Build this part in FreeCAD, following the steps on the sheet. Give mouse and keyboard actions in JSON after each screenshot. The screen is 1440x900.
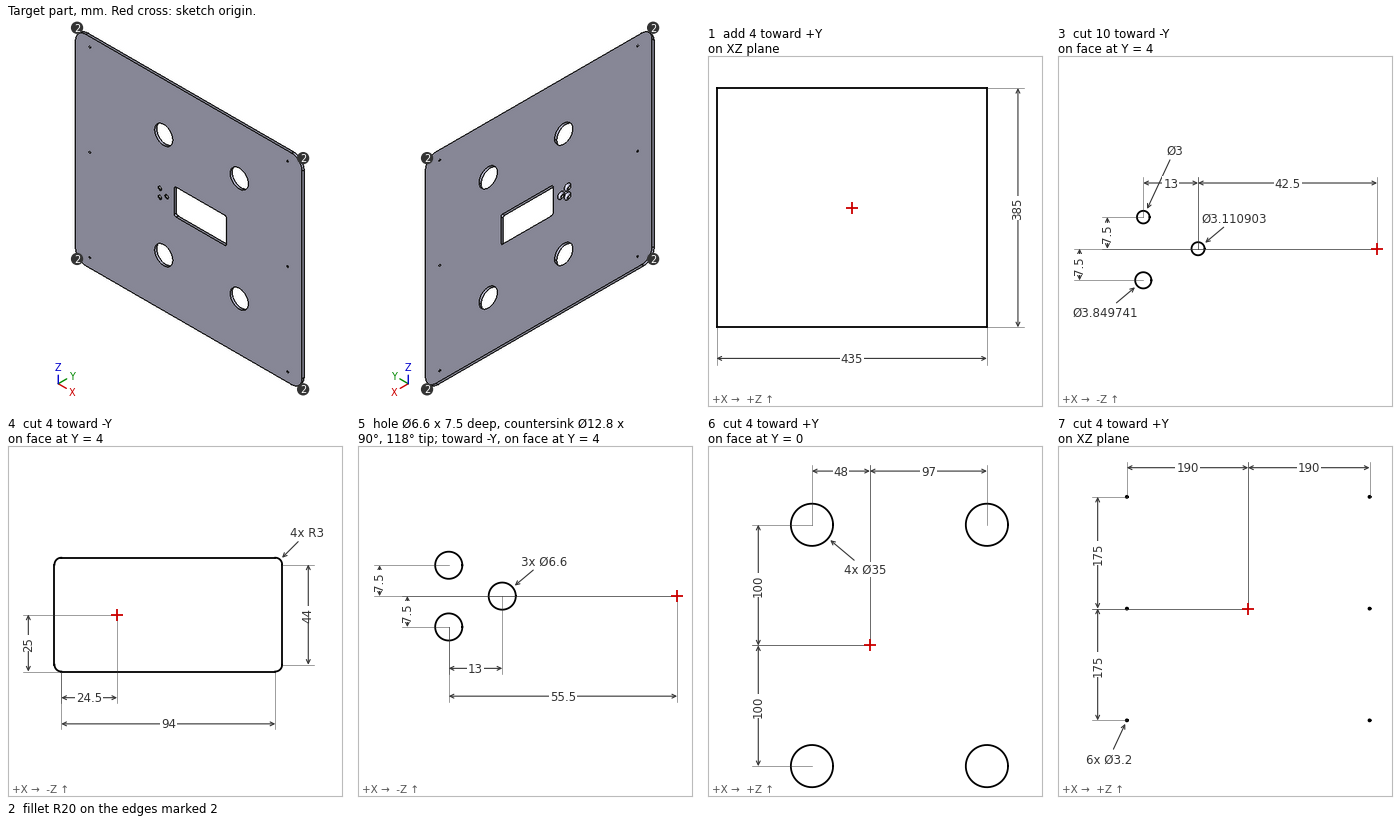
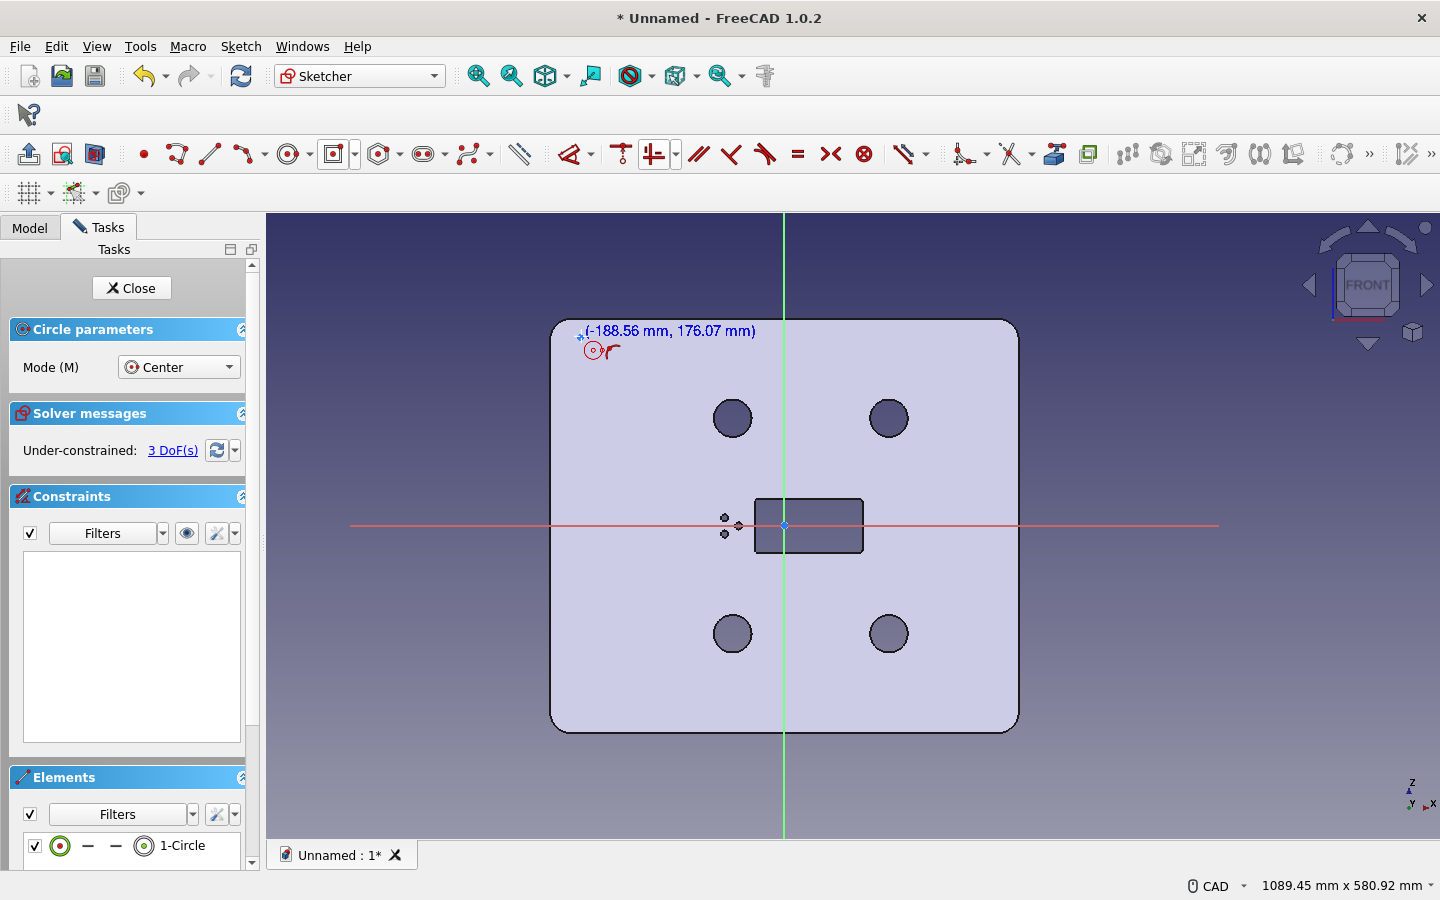
{"action": "scroll", "coordinate": [580, 526], "scroll_direction": "up", "scroll_amount": 13}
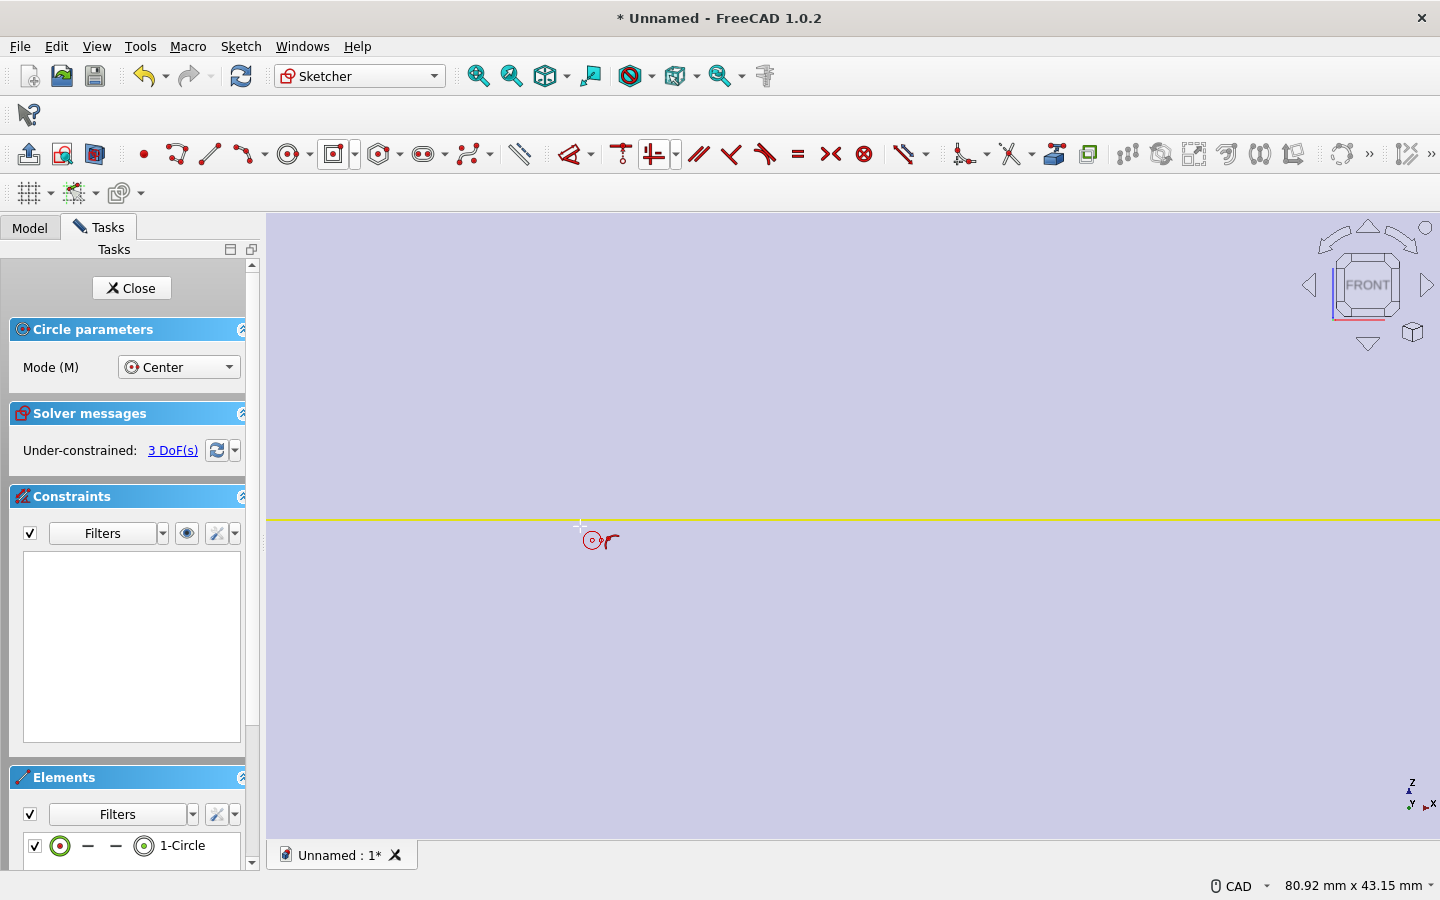
{"action": "scroll", "coordinate": [580, 527], "scroll_direction": "down", "scroll_amount": 13}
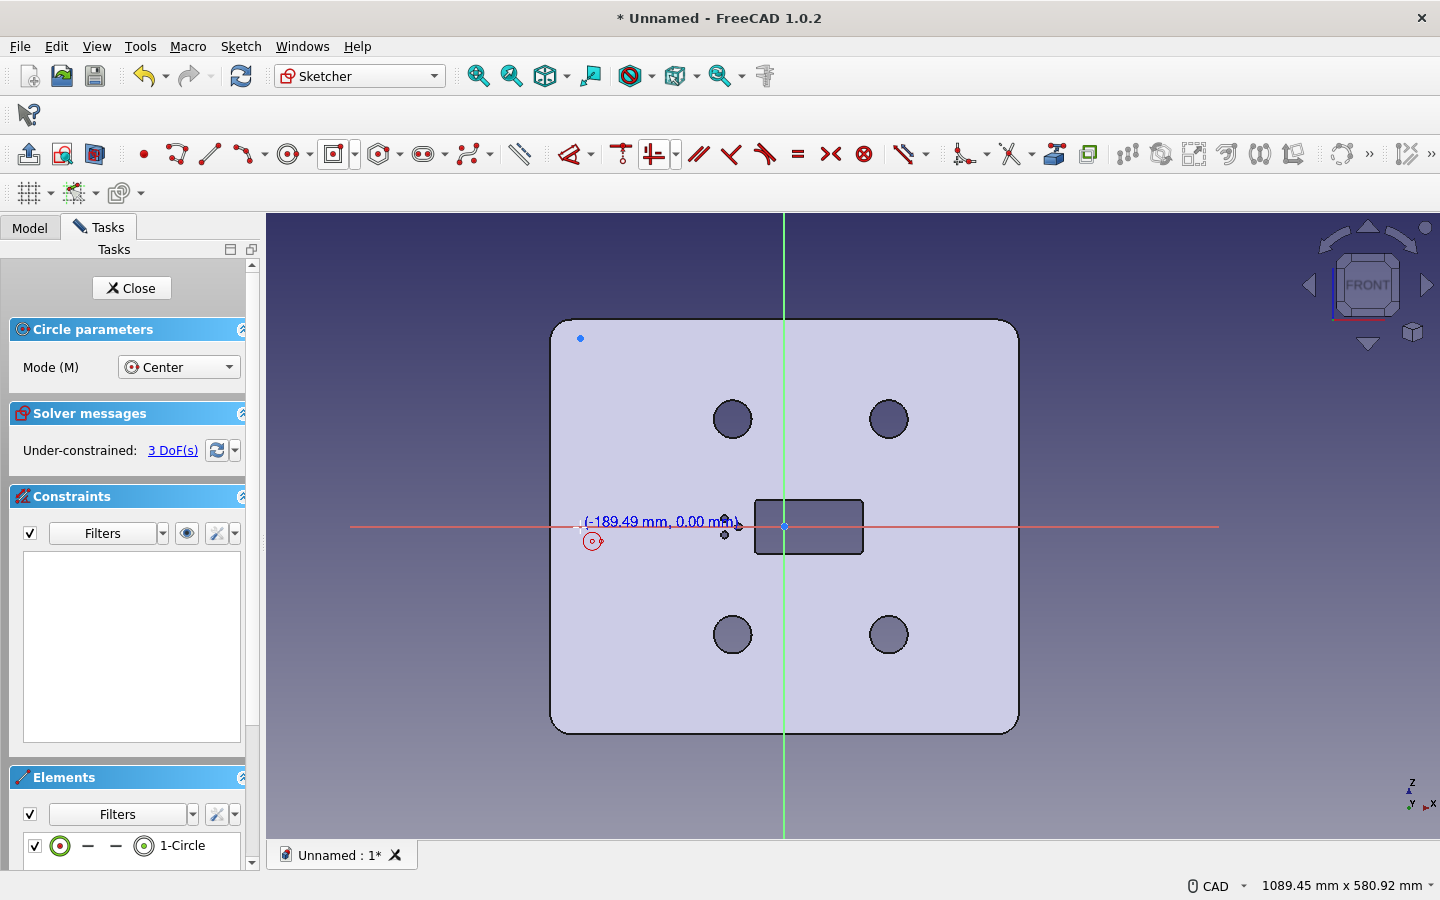
{"action": "left_click", "coordinate": [580, 527]}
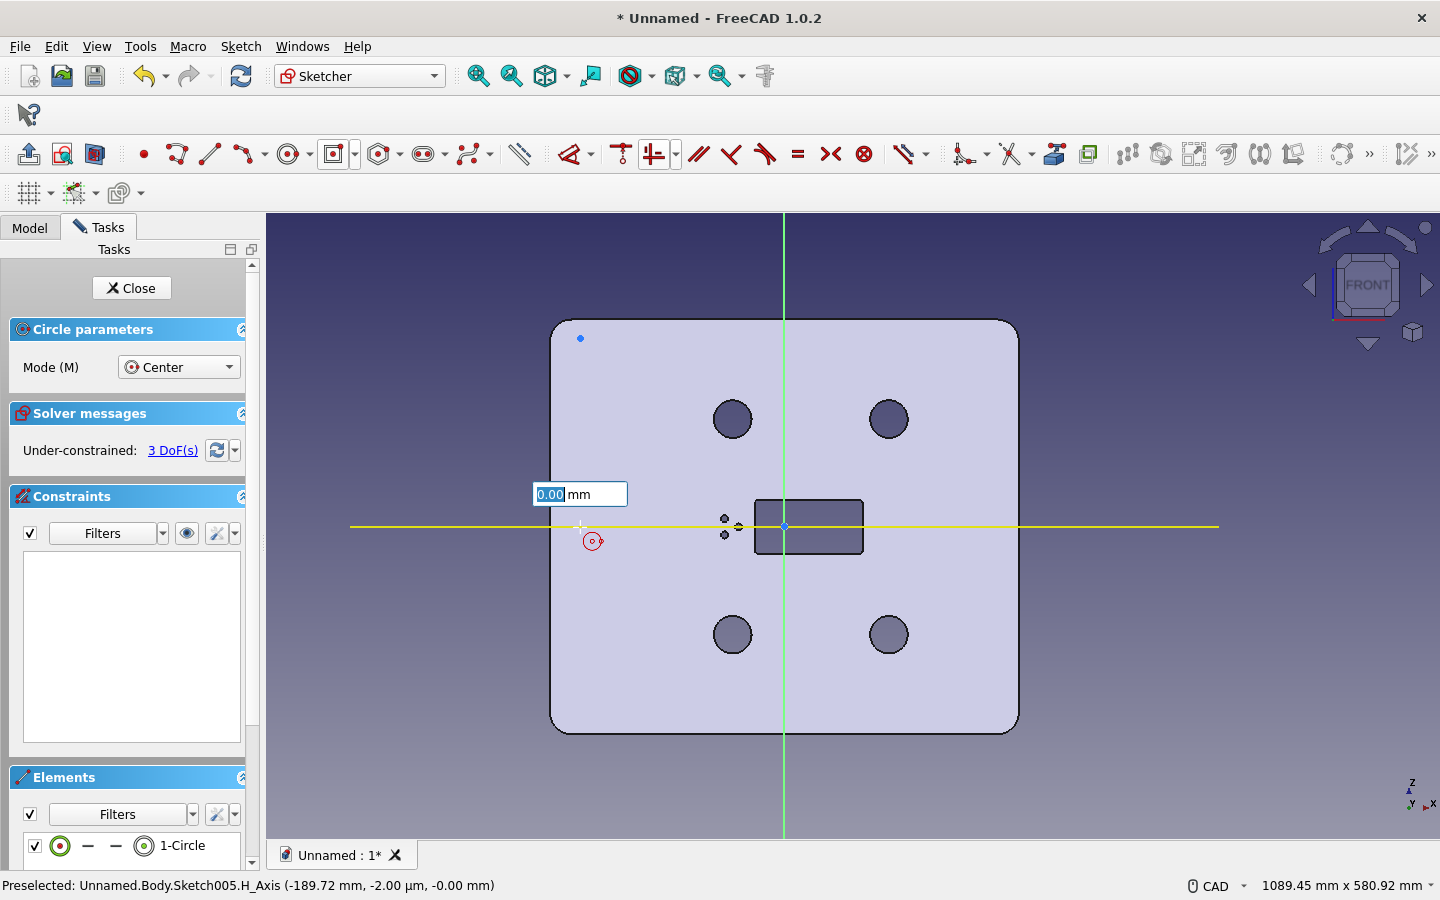
{"action": "scroll", "coordinate": [579, 529], "scroll_direction": "up", "scroll_amount": 12}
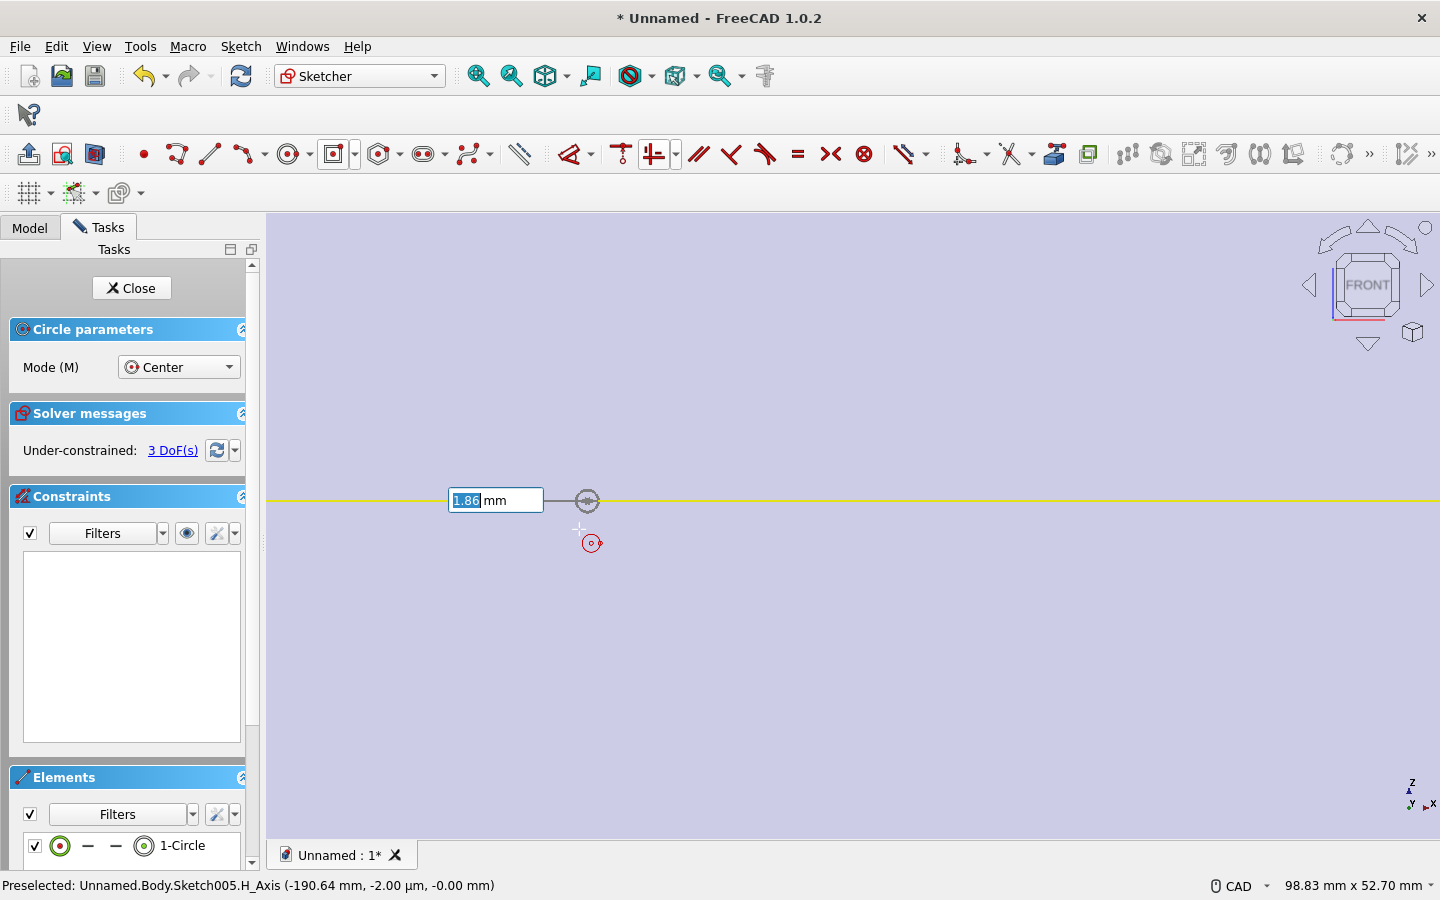
{"action": "left_click", "coordinate": [577, 519]}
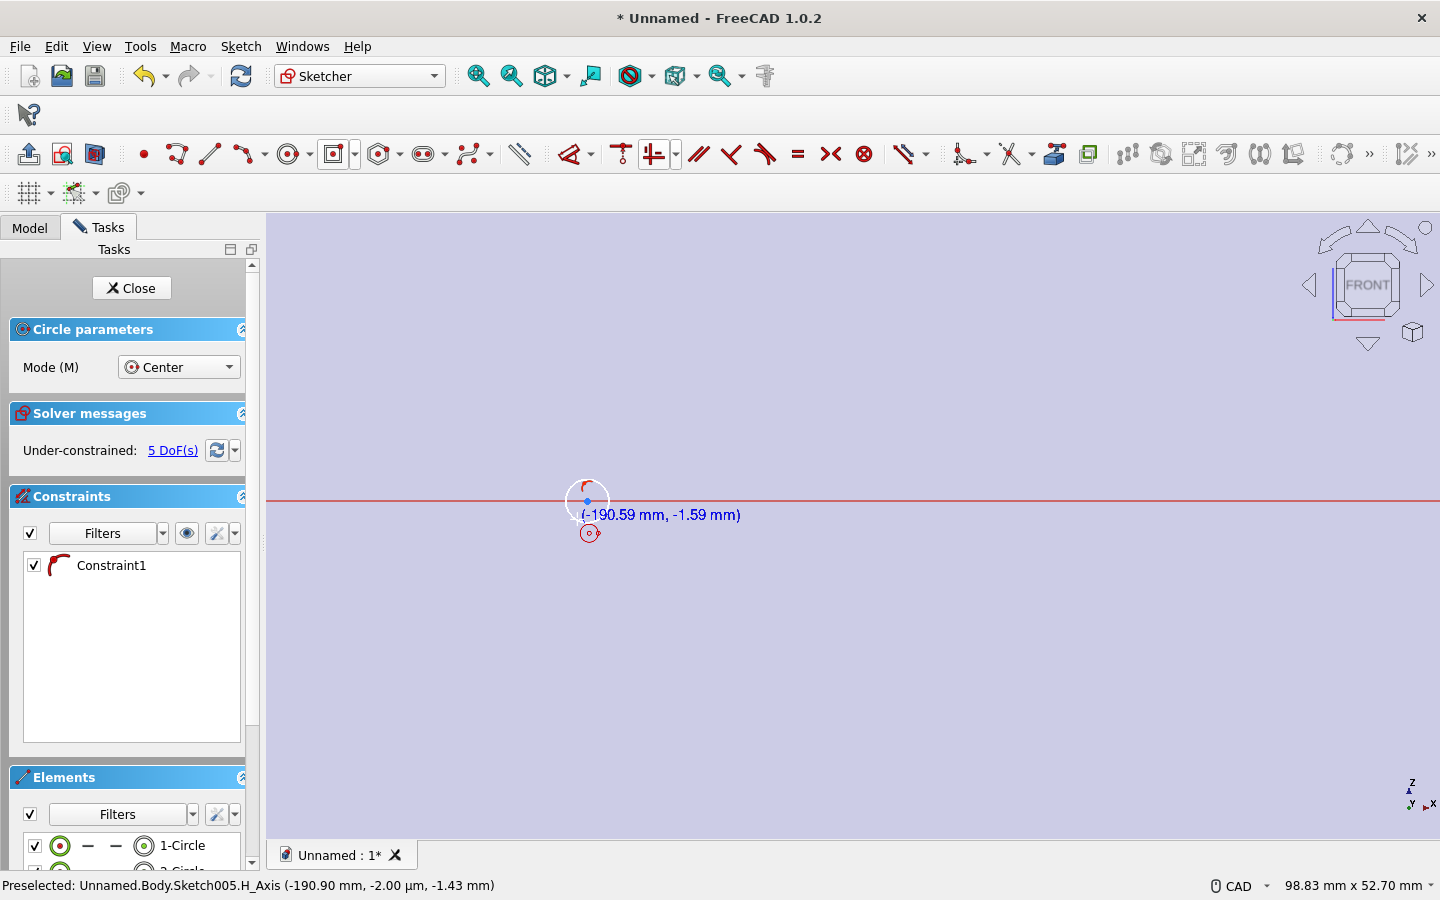
{"action": "scroll", "coordinate": [579, 528], "scroll_direction": "down", "scroll_amount": 12}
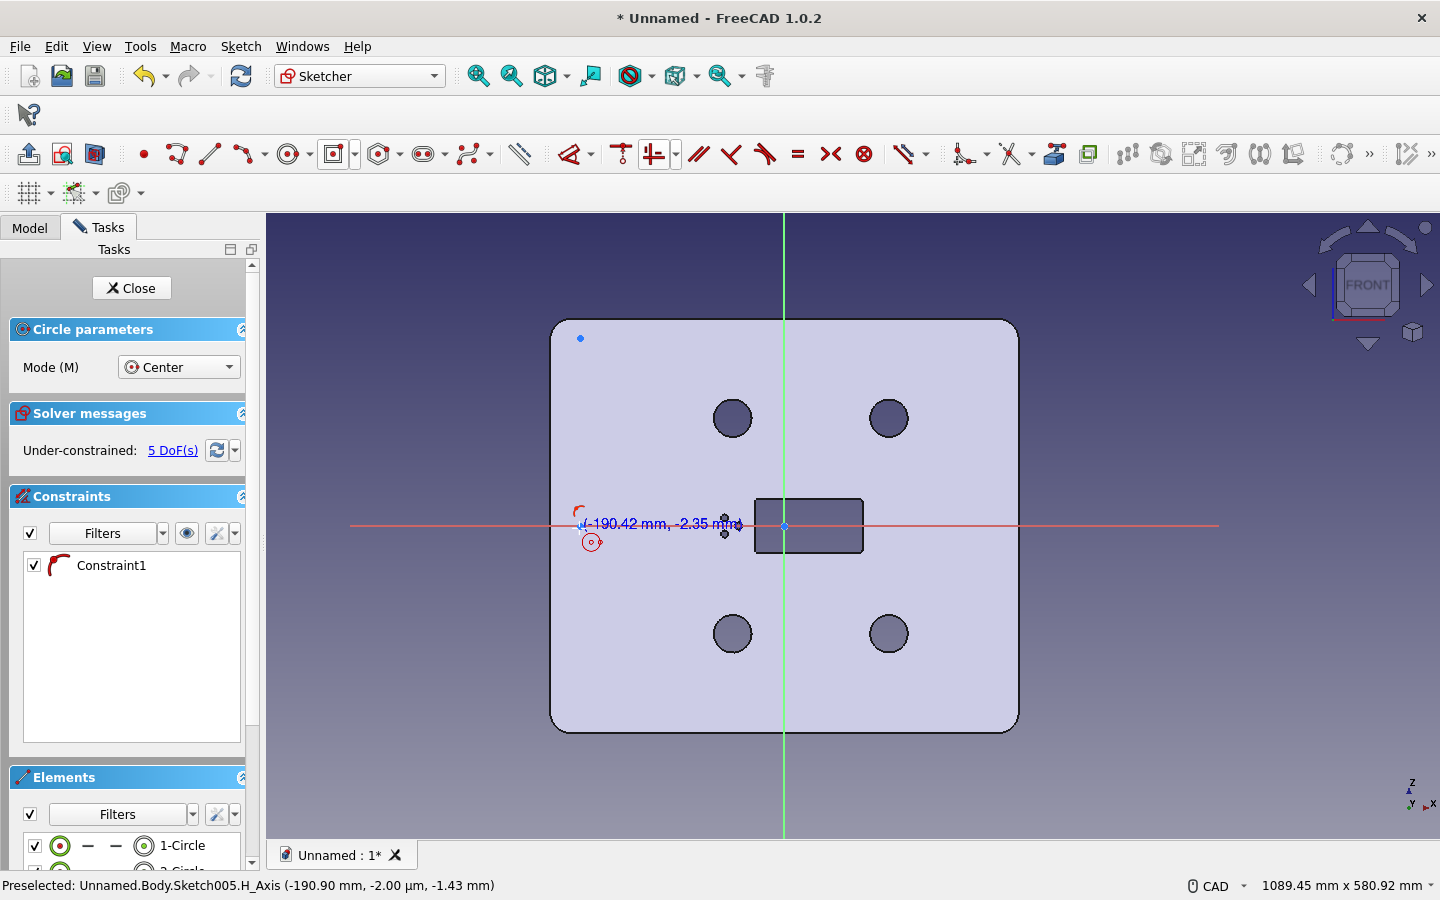
{"action": "scroll", "coordinate": [580, 715], "scroll_direction": "up", "scroll_amount": 13}